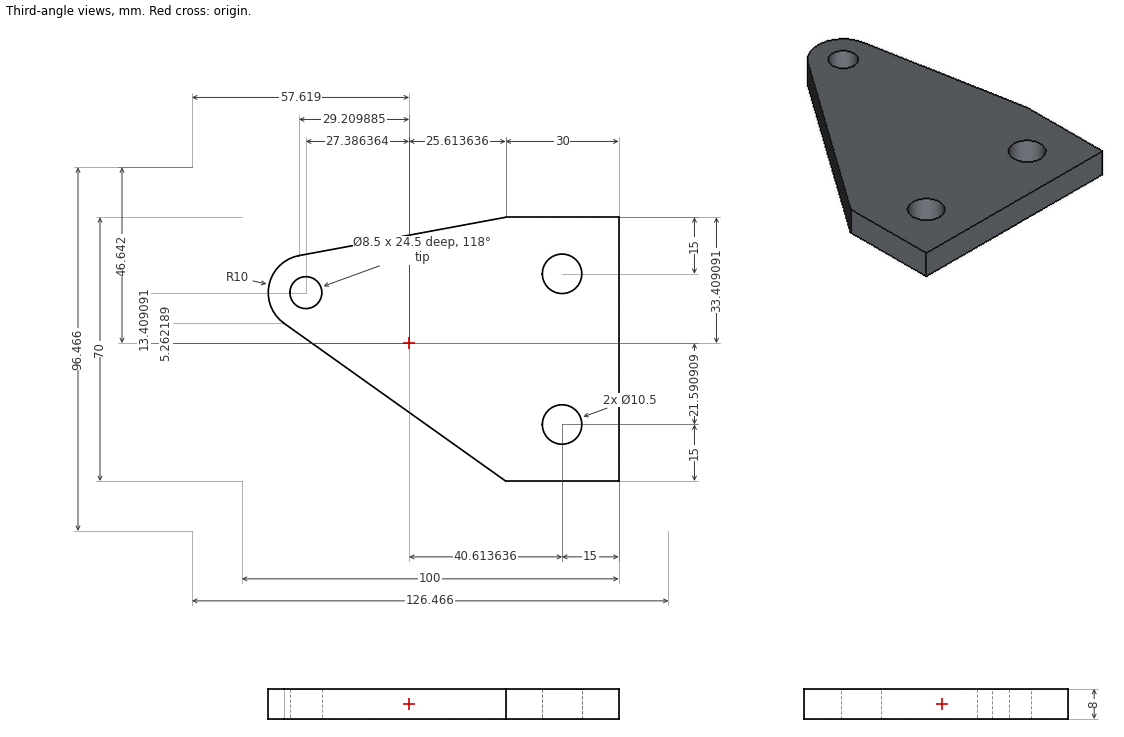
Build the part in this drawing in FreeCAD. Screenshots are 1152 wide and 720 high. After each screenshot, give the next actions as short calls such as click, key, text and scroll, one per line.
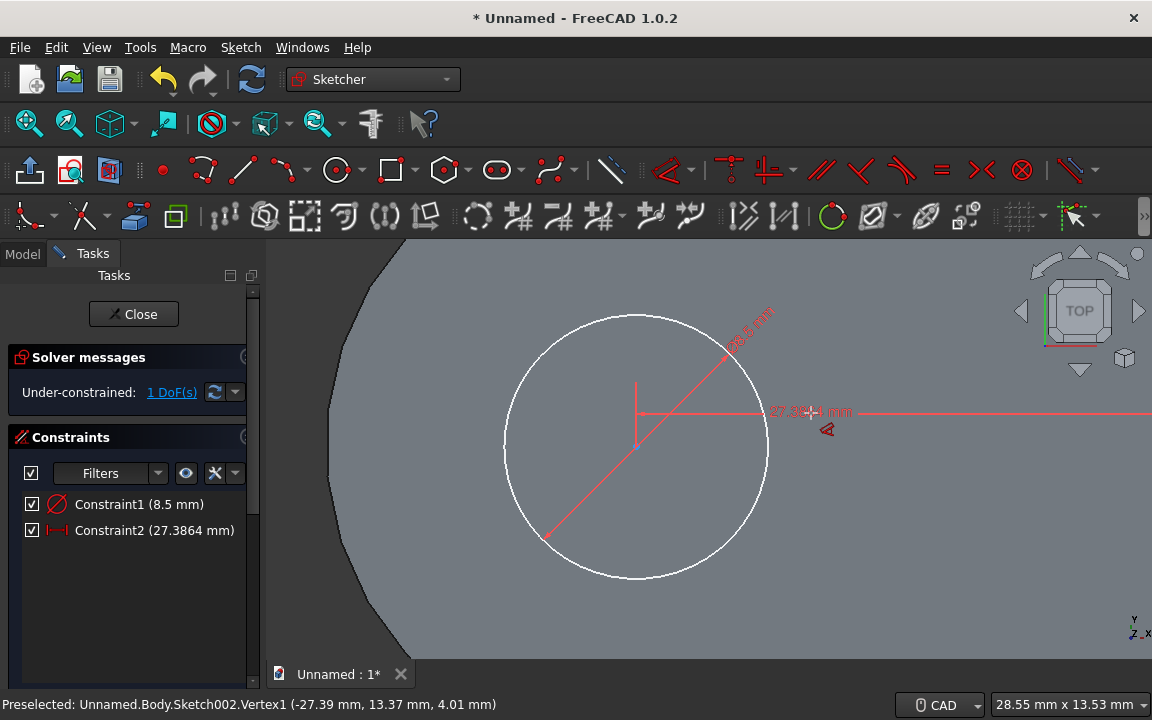
click(636, 447)
click(602, 539)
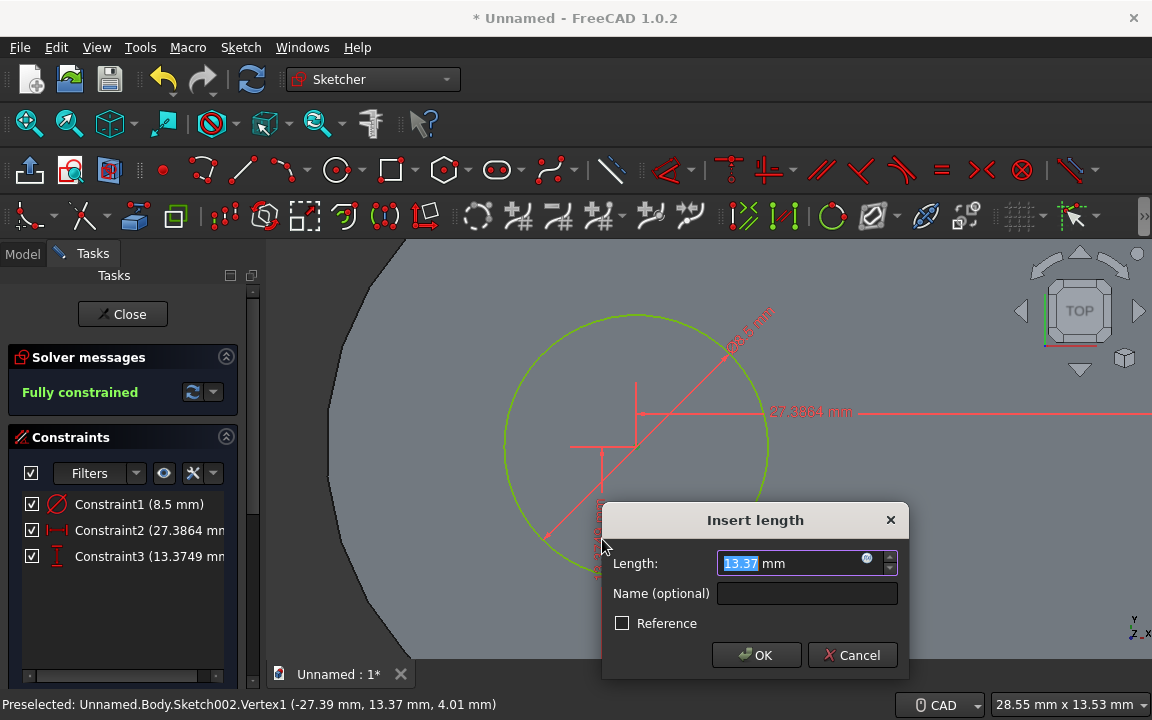
text(13.409091)
key(Return)
key(Escape)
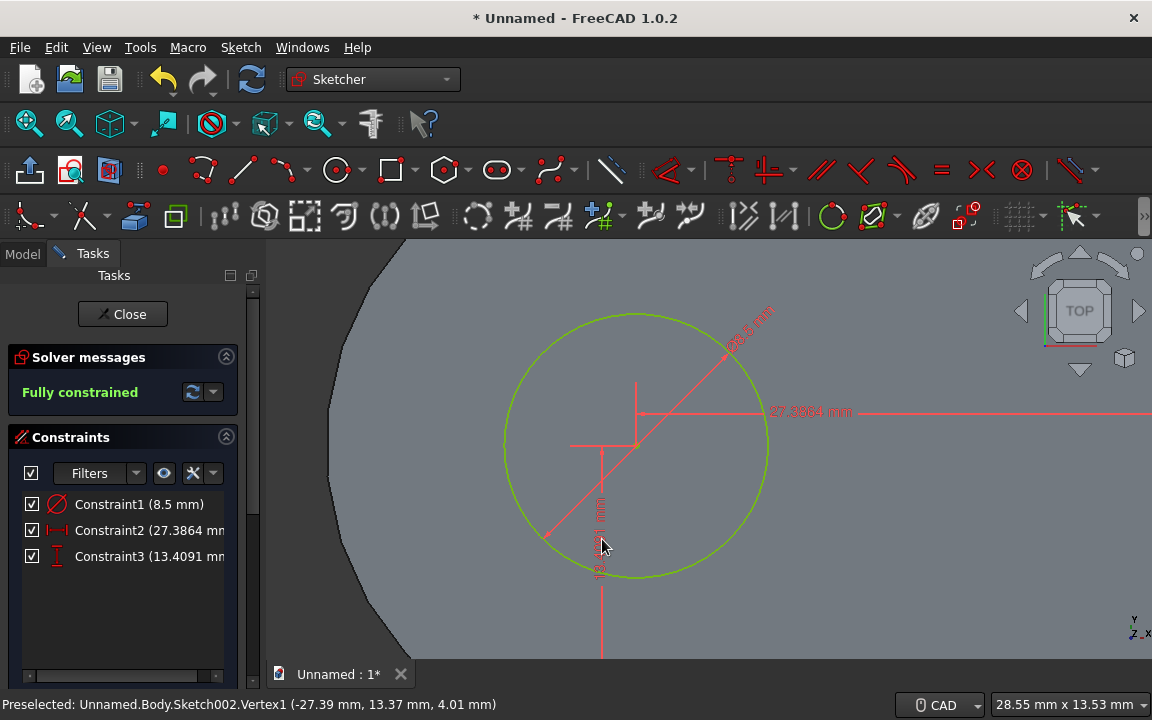
click(123, 314)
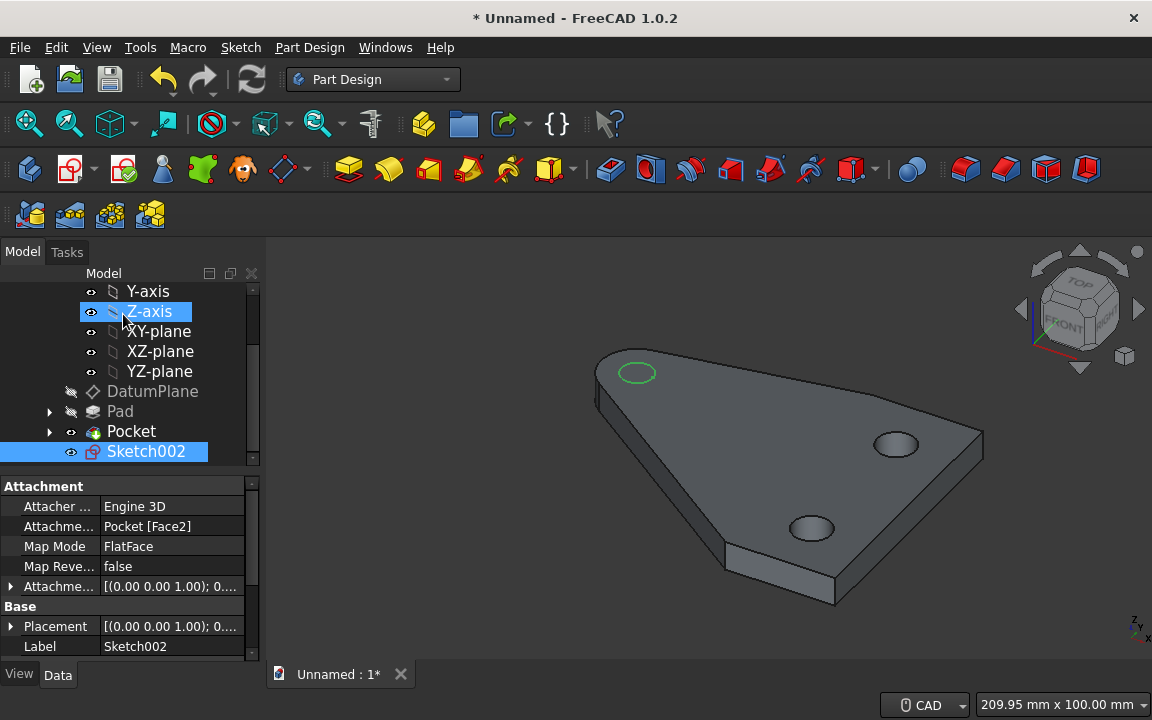
click(652, 170)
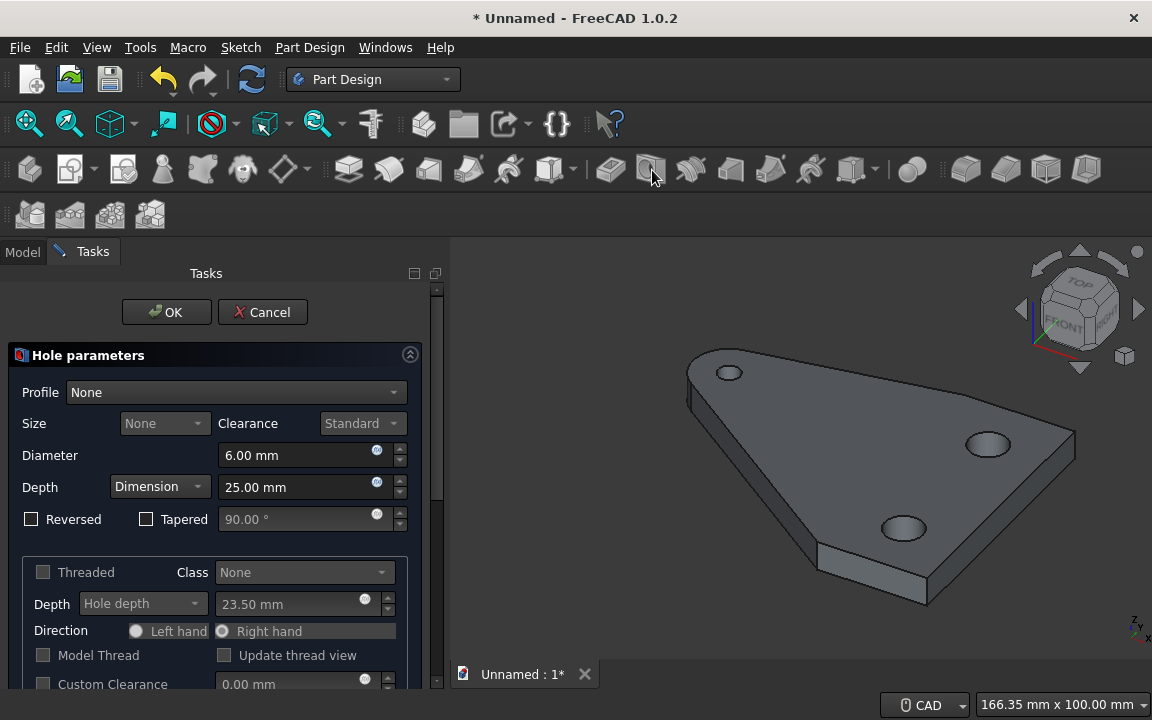
triple_click(305, 455)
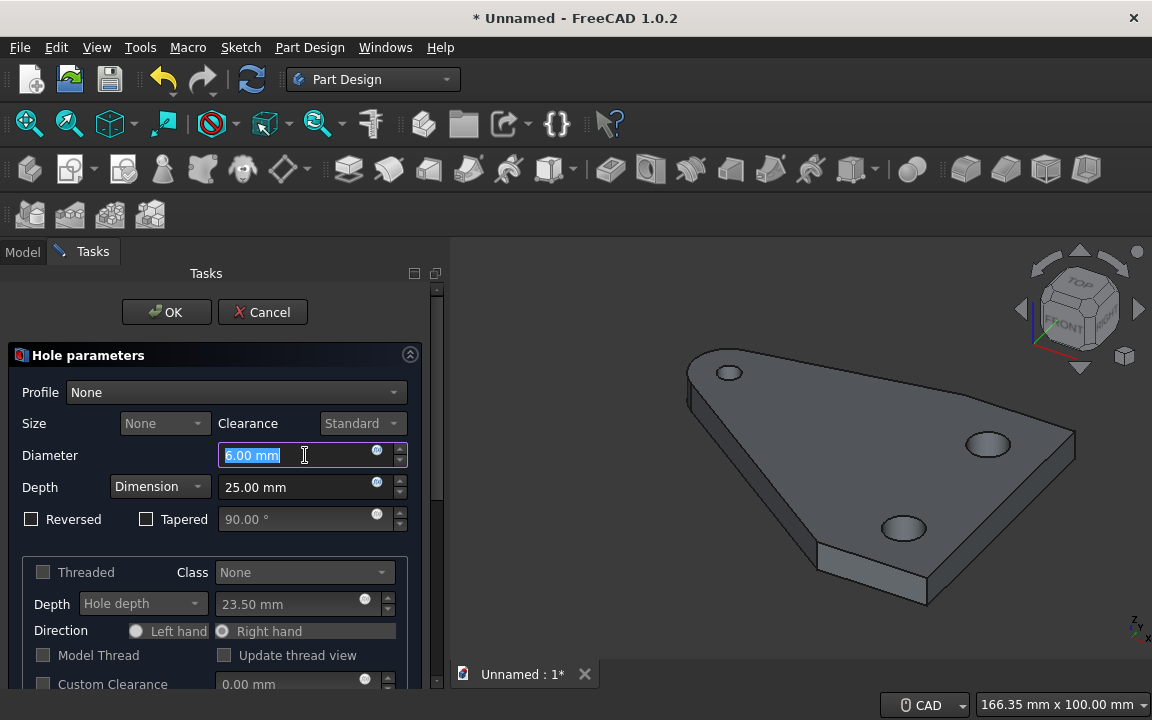
text(8.5)
key(Tab)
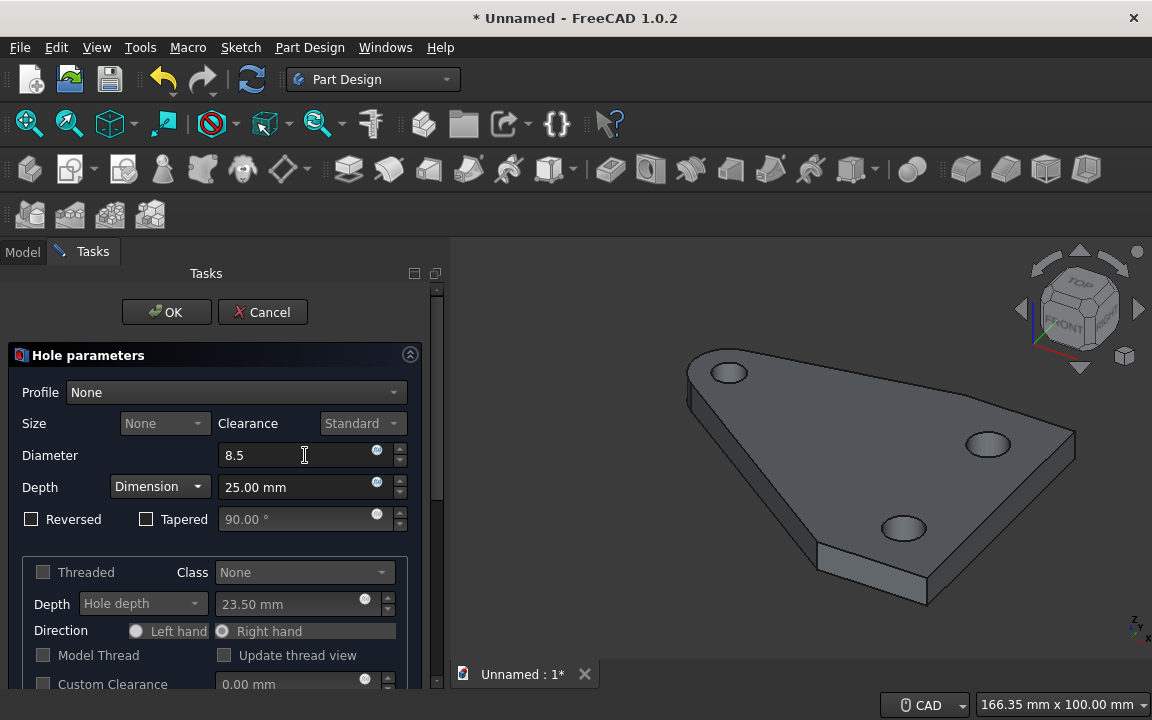
triple_click(305, 487)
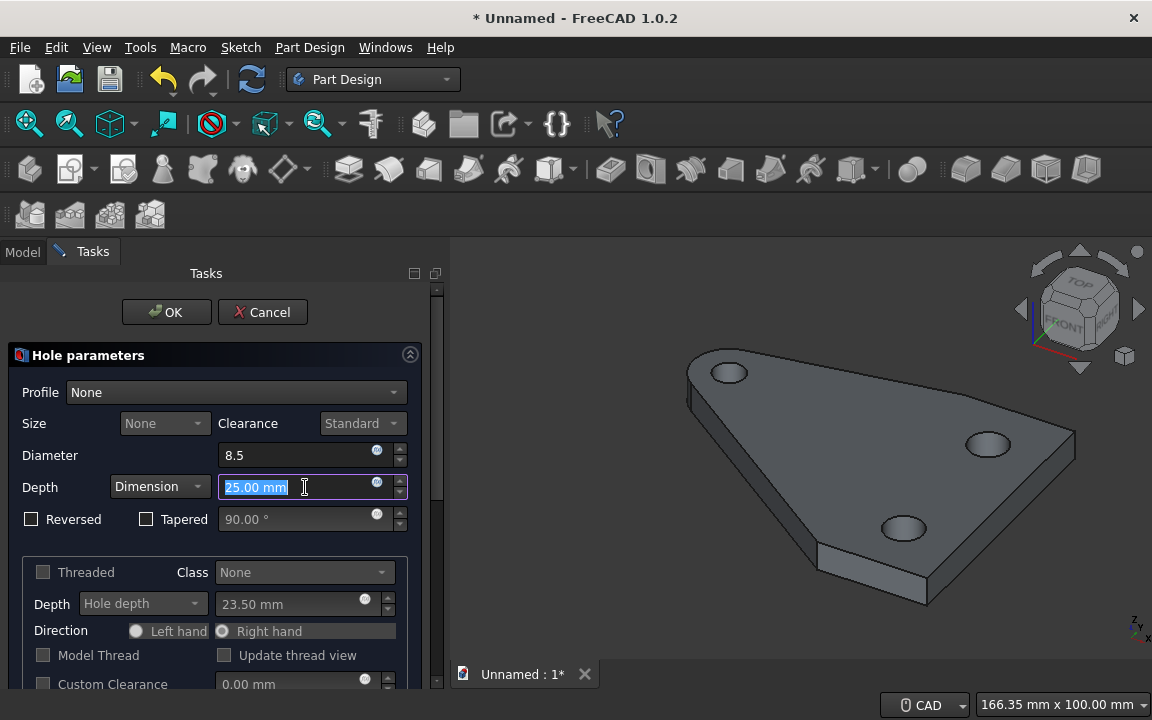
text(24.5)
key(Tab)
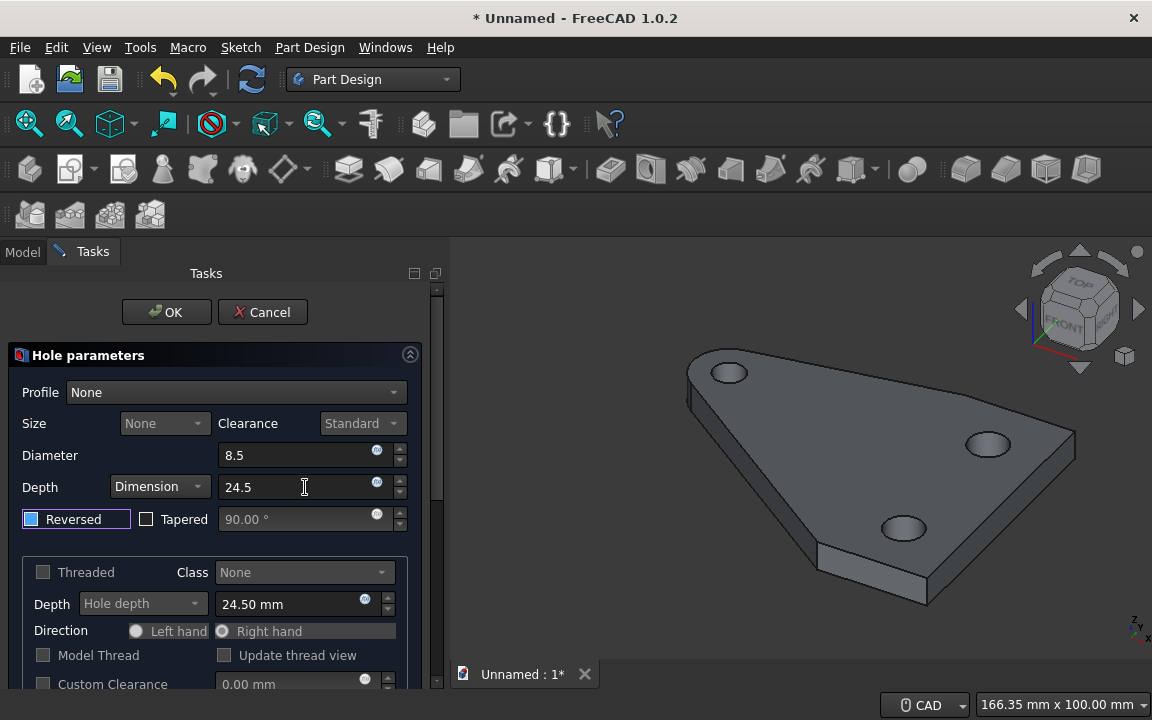
click(167, 312)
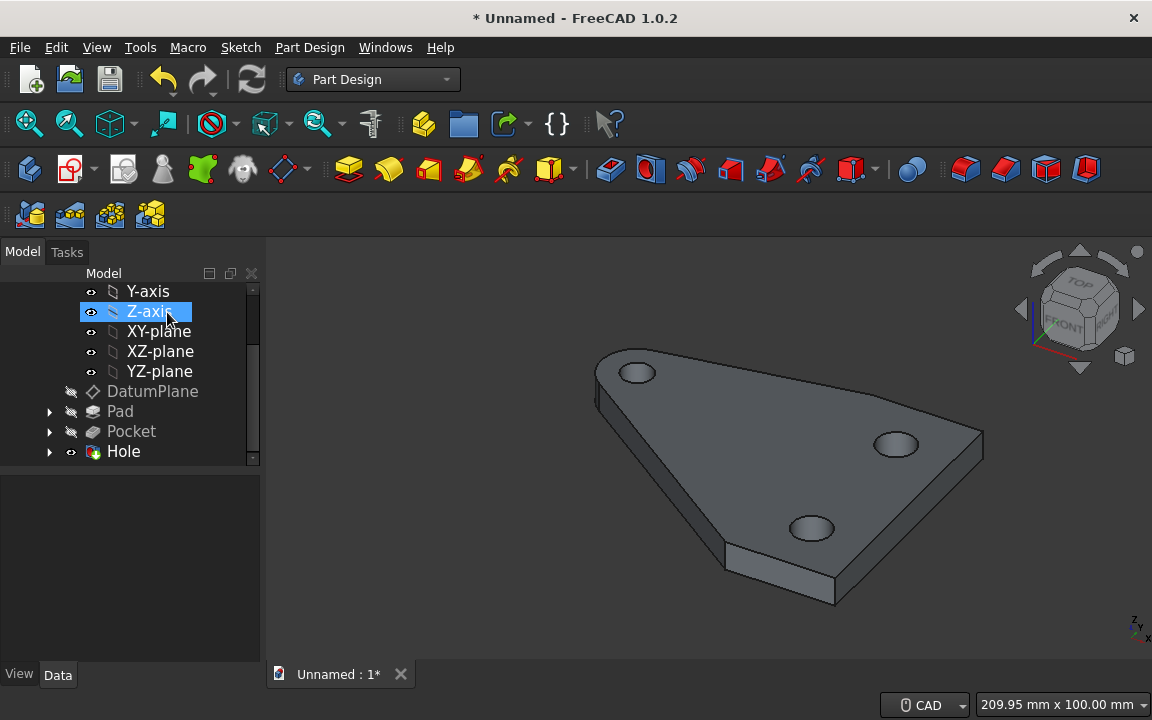
key(0)